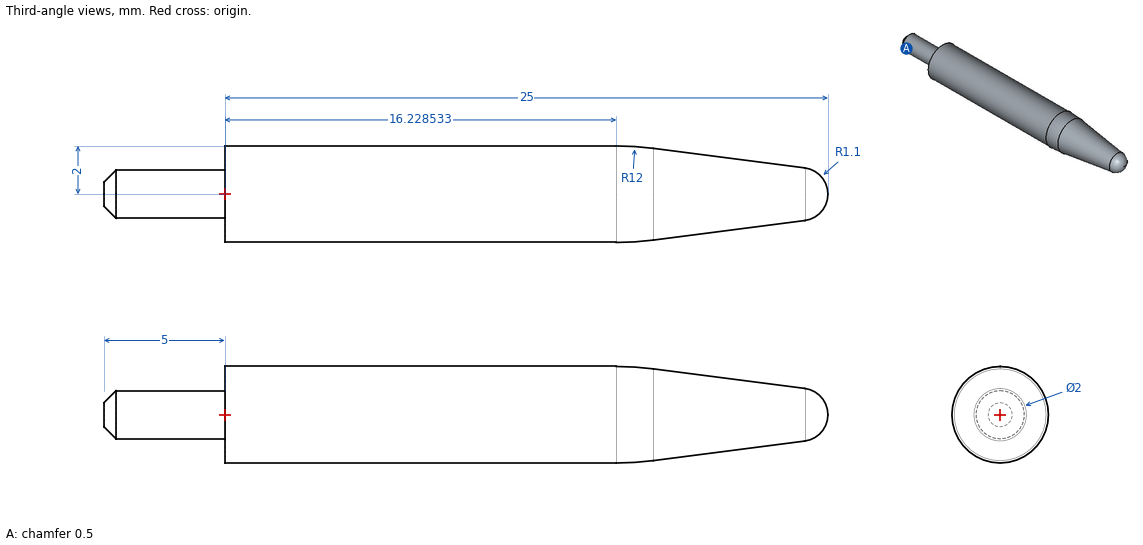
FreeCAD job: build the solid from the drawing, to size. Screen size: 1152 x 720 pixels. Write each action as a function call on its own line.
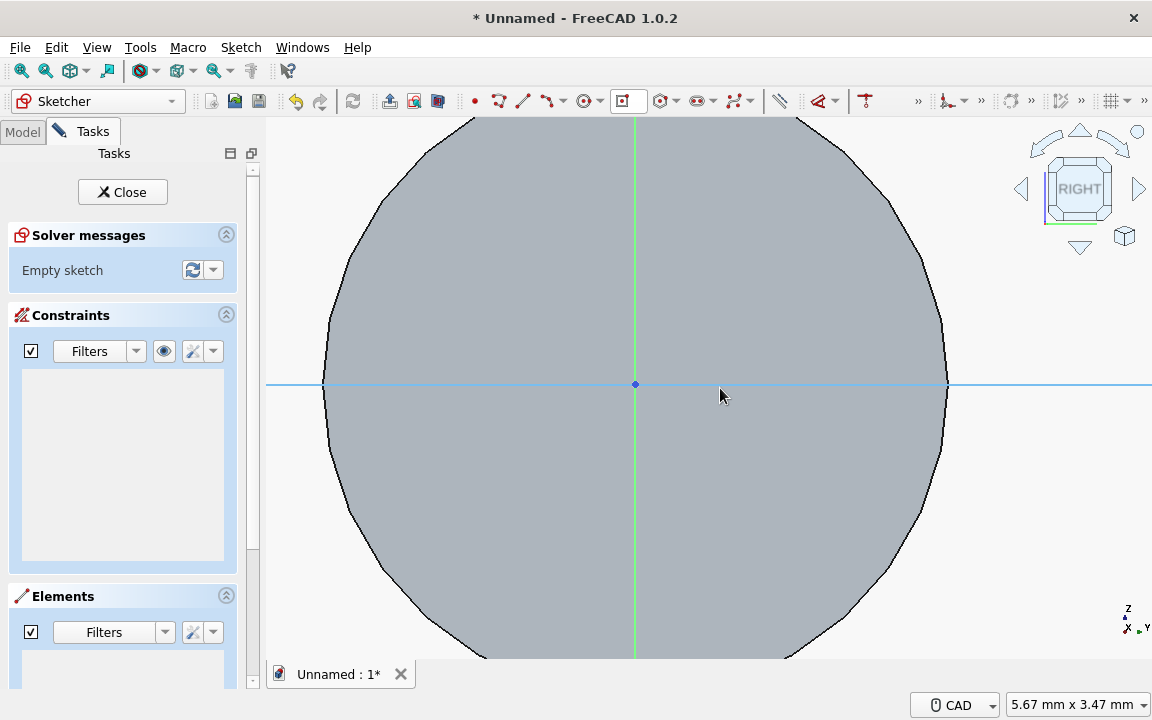
key(g)
key(c)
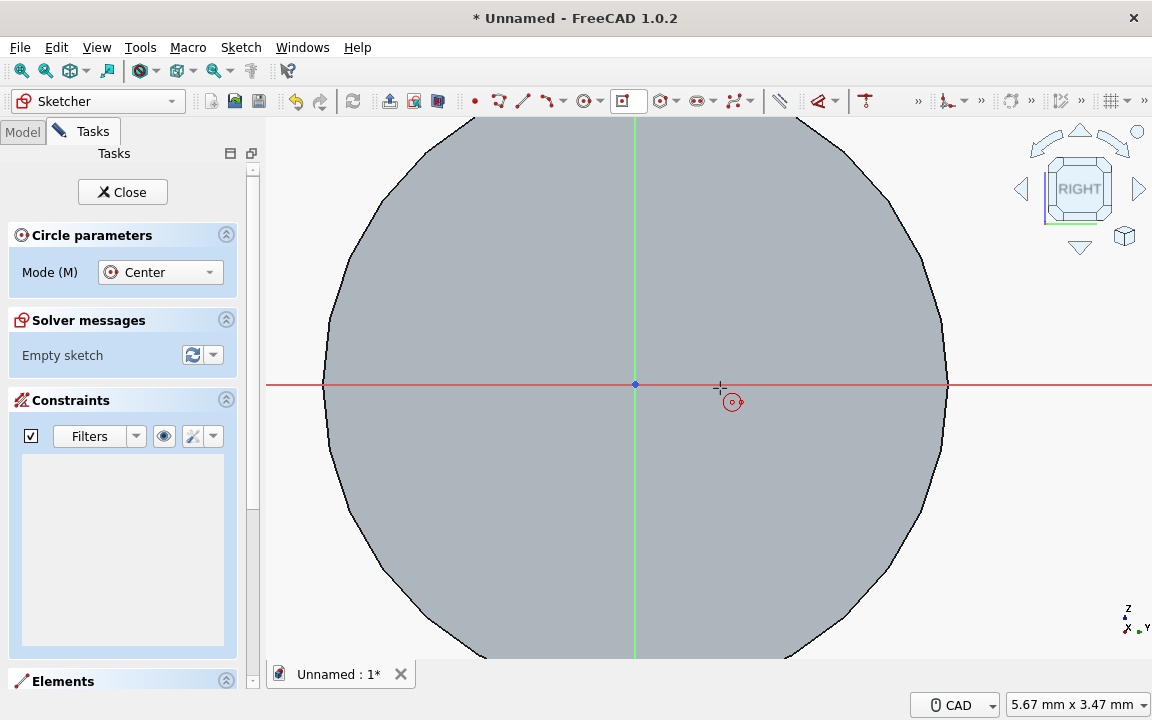
click(635, 385)
click(746, 274)
key(Escape)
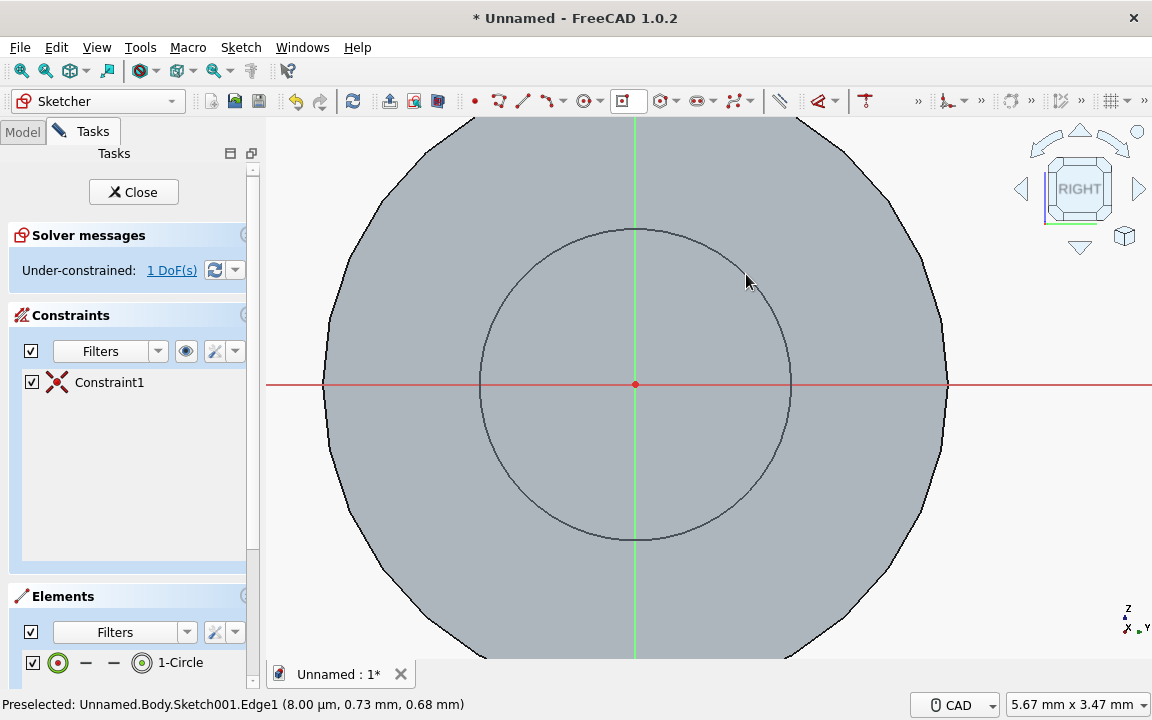
click(818, 102)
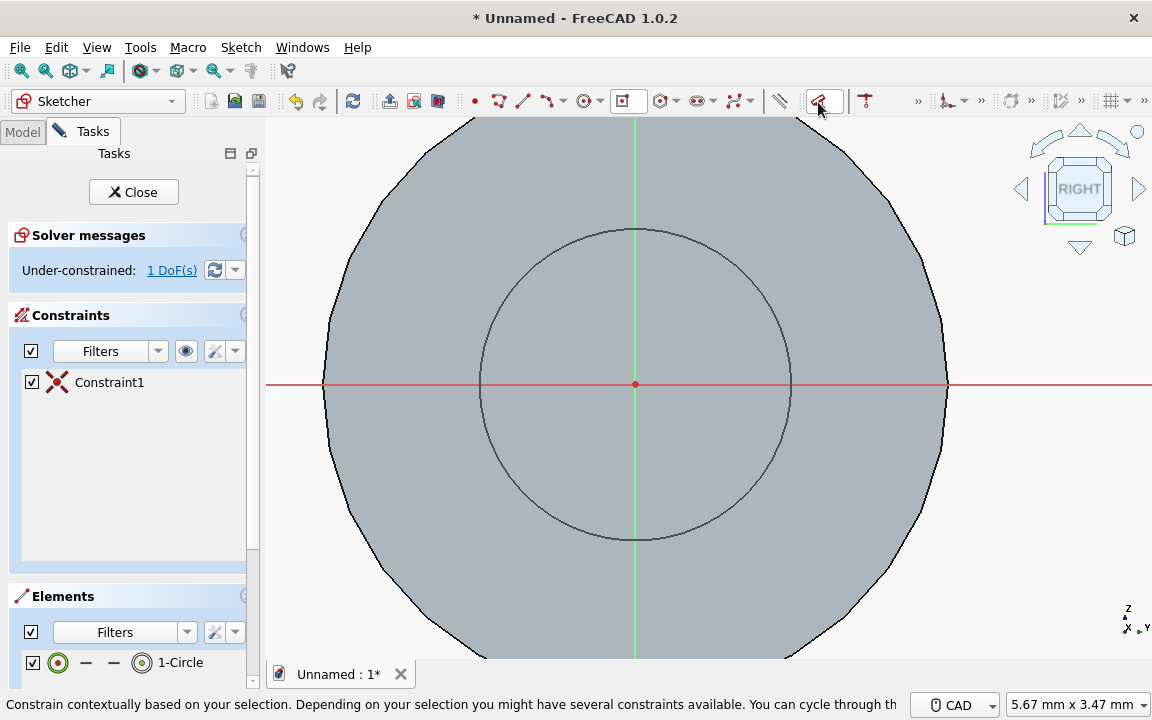
click(745, 274)
click(767, 251)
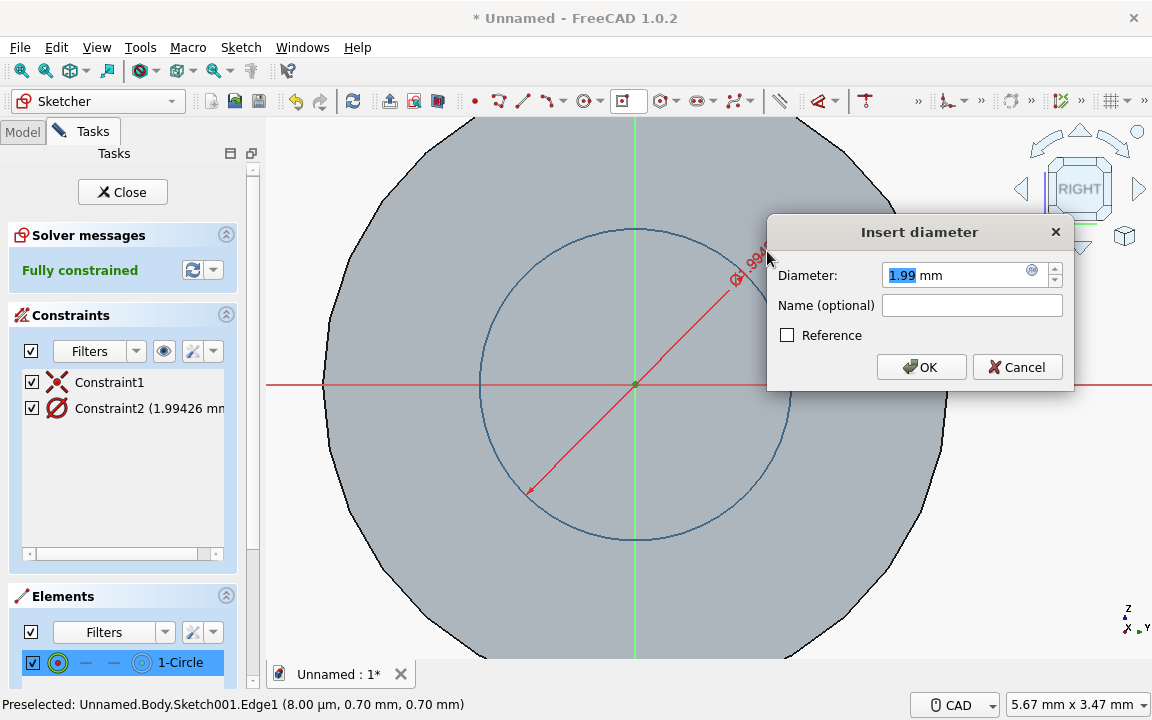
text(2)
key(Return)
key(Escape)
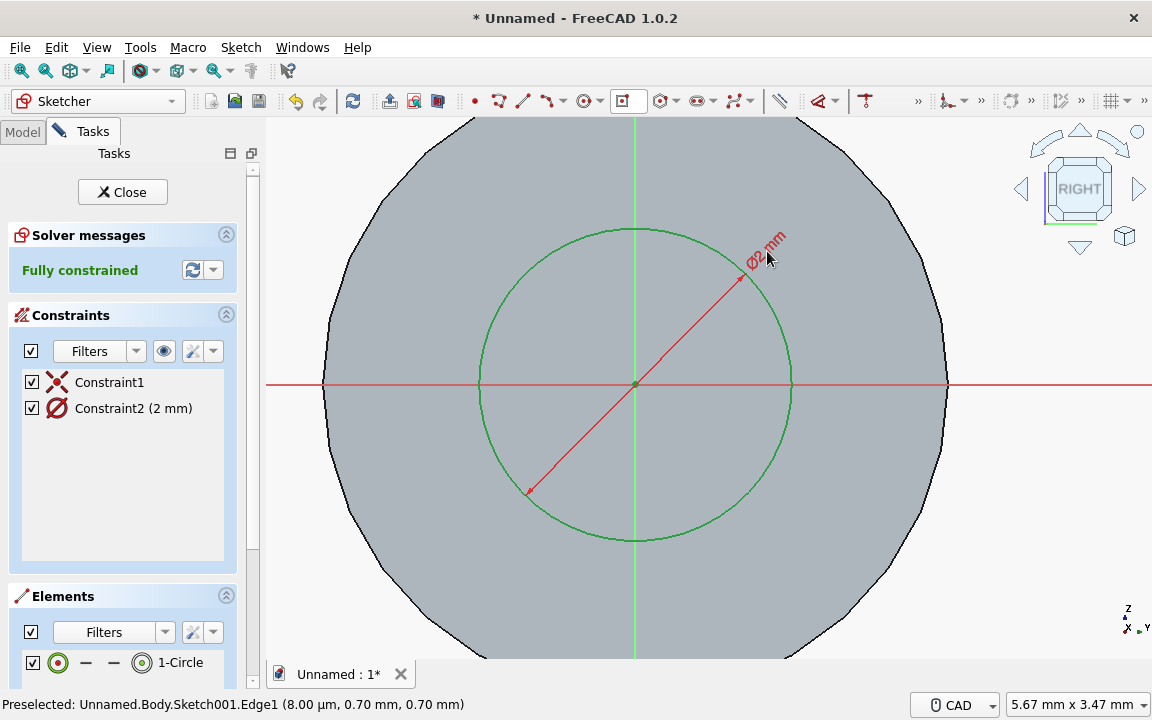
click(123, 192)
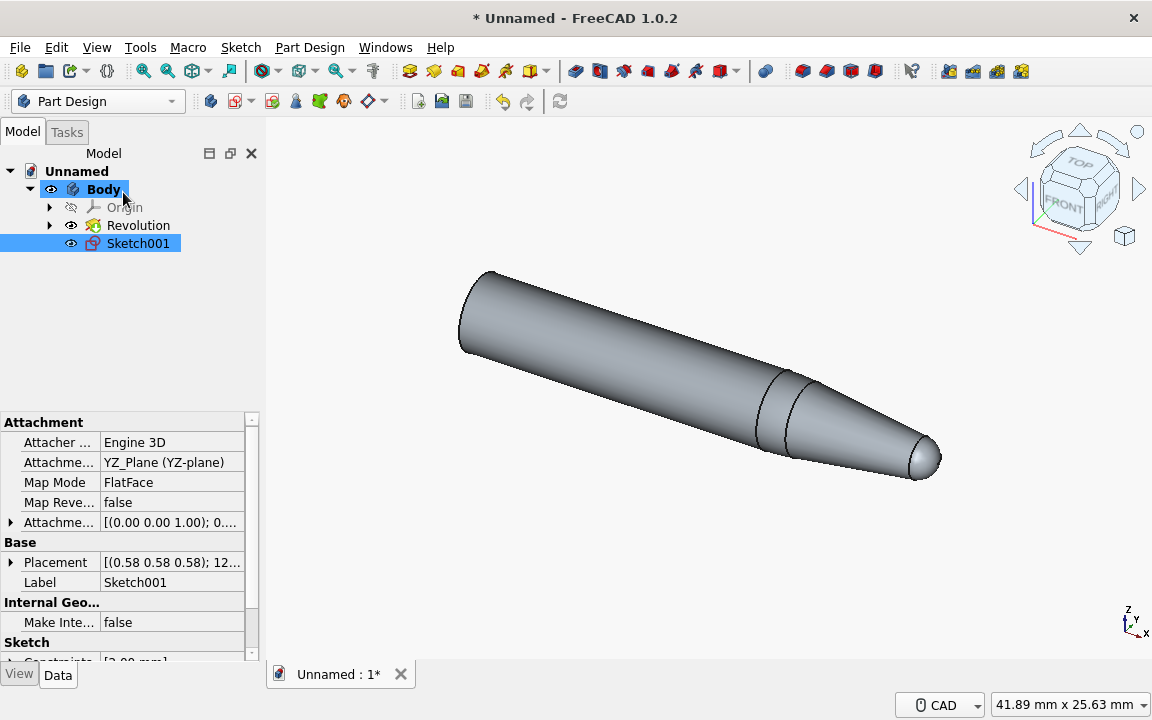
click(410, 72)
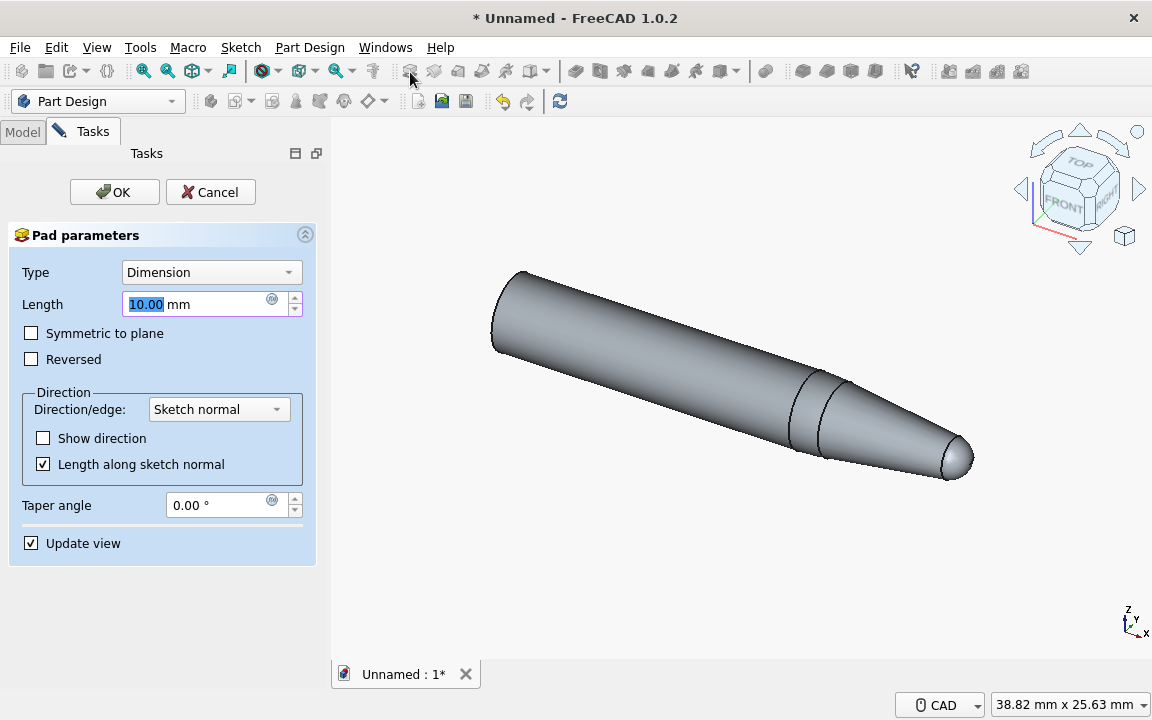
text(5)
key(Tab)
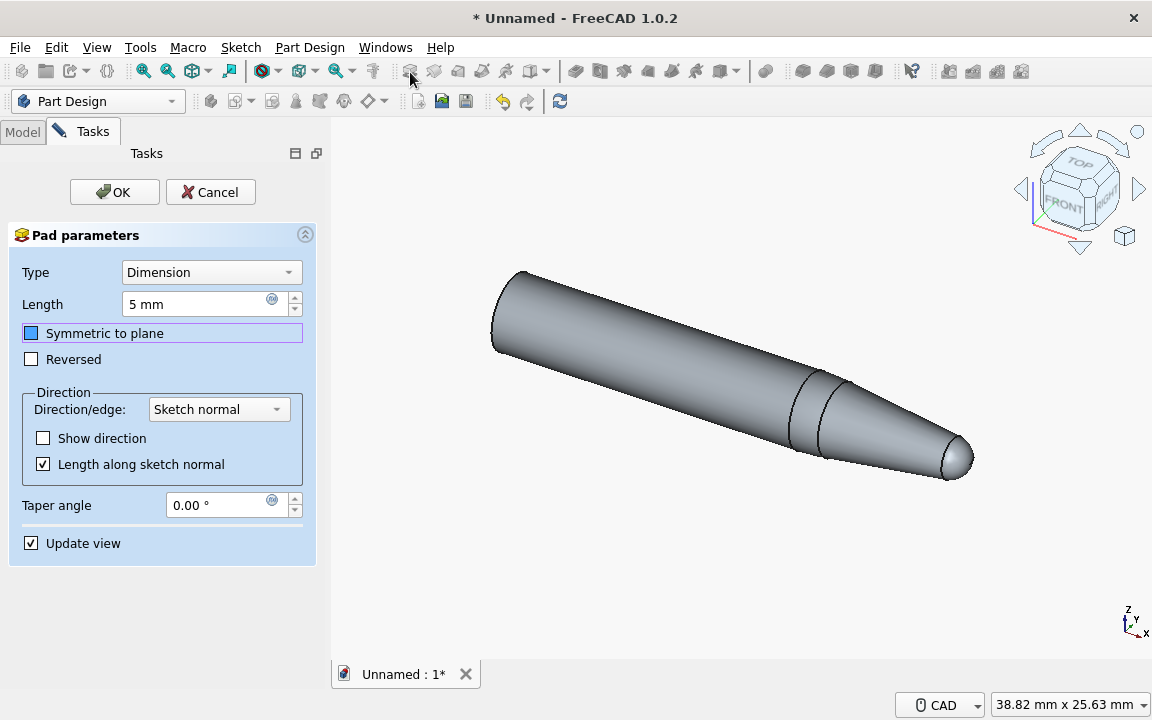
click(30, 359)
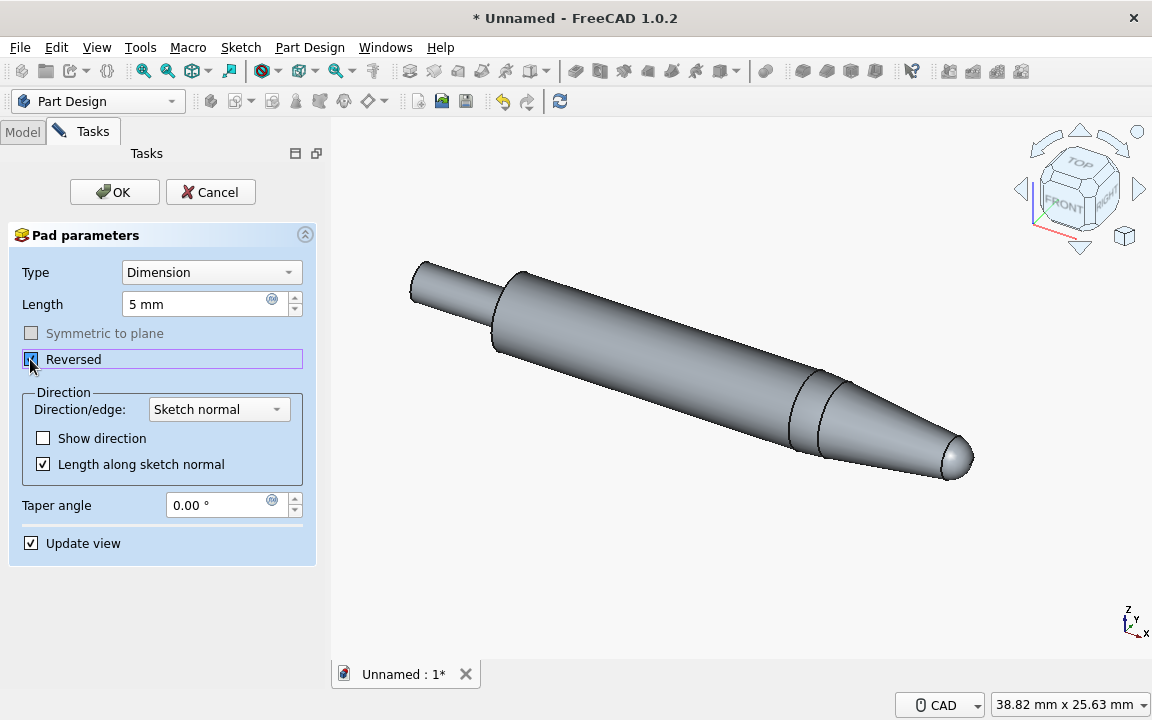
click(115, 192)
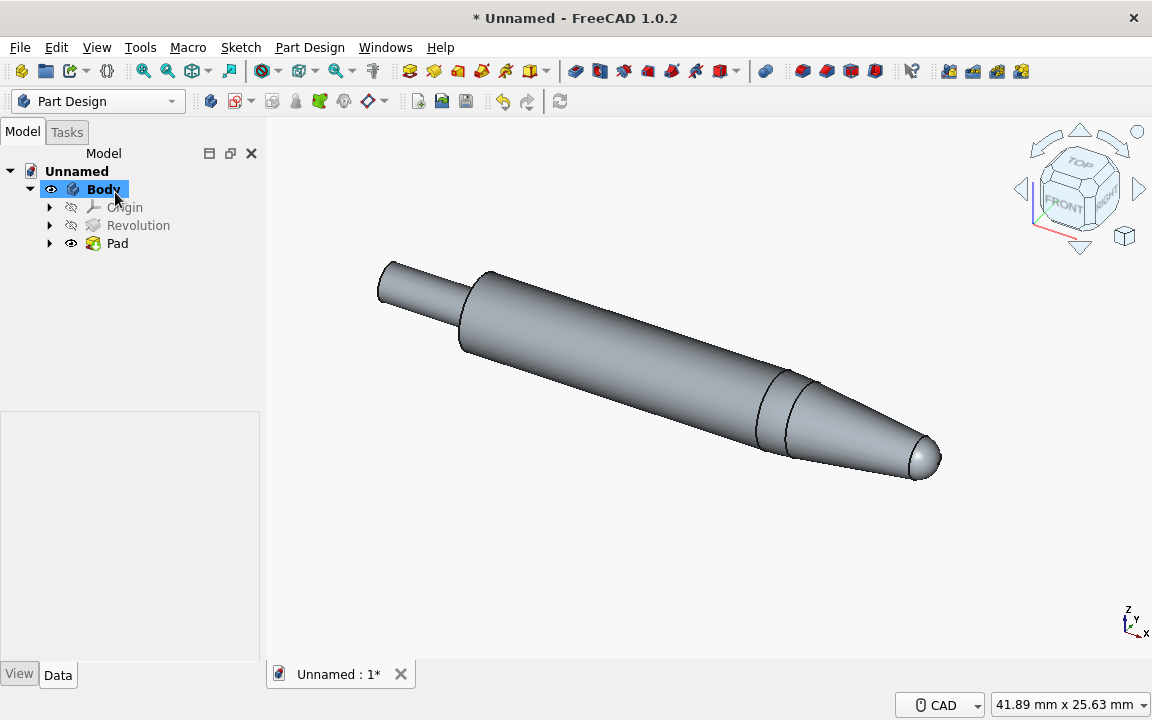
click(392, 261)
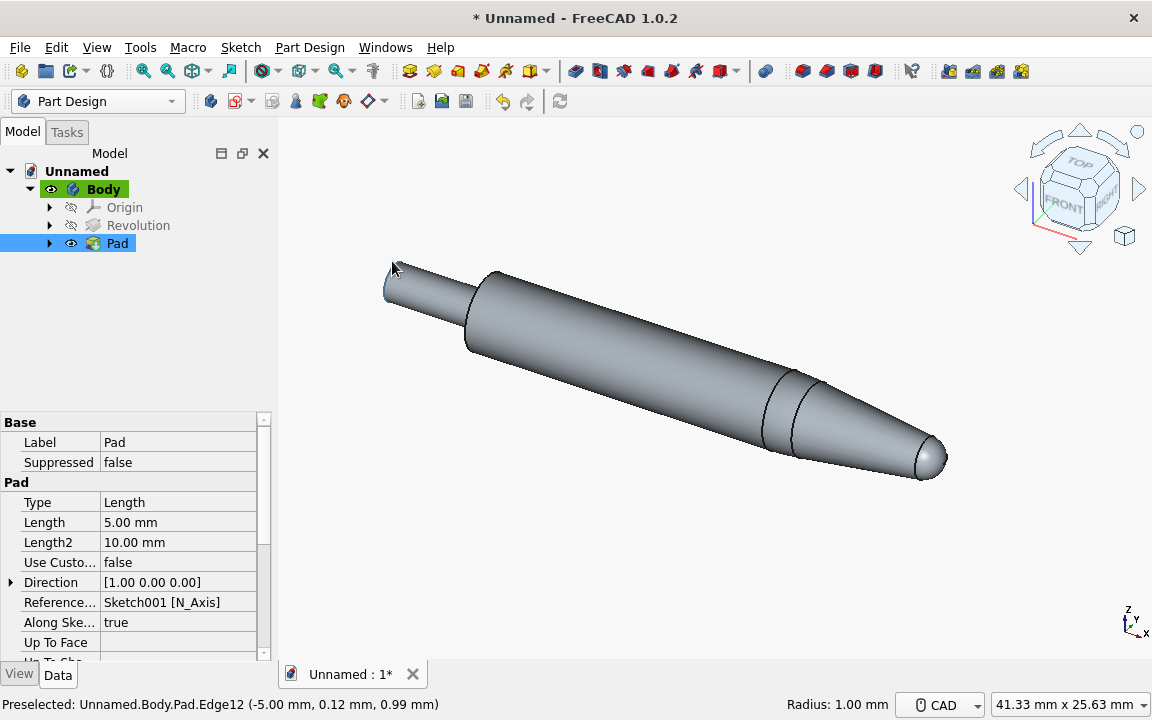
click(828, 72)